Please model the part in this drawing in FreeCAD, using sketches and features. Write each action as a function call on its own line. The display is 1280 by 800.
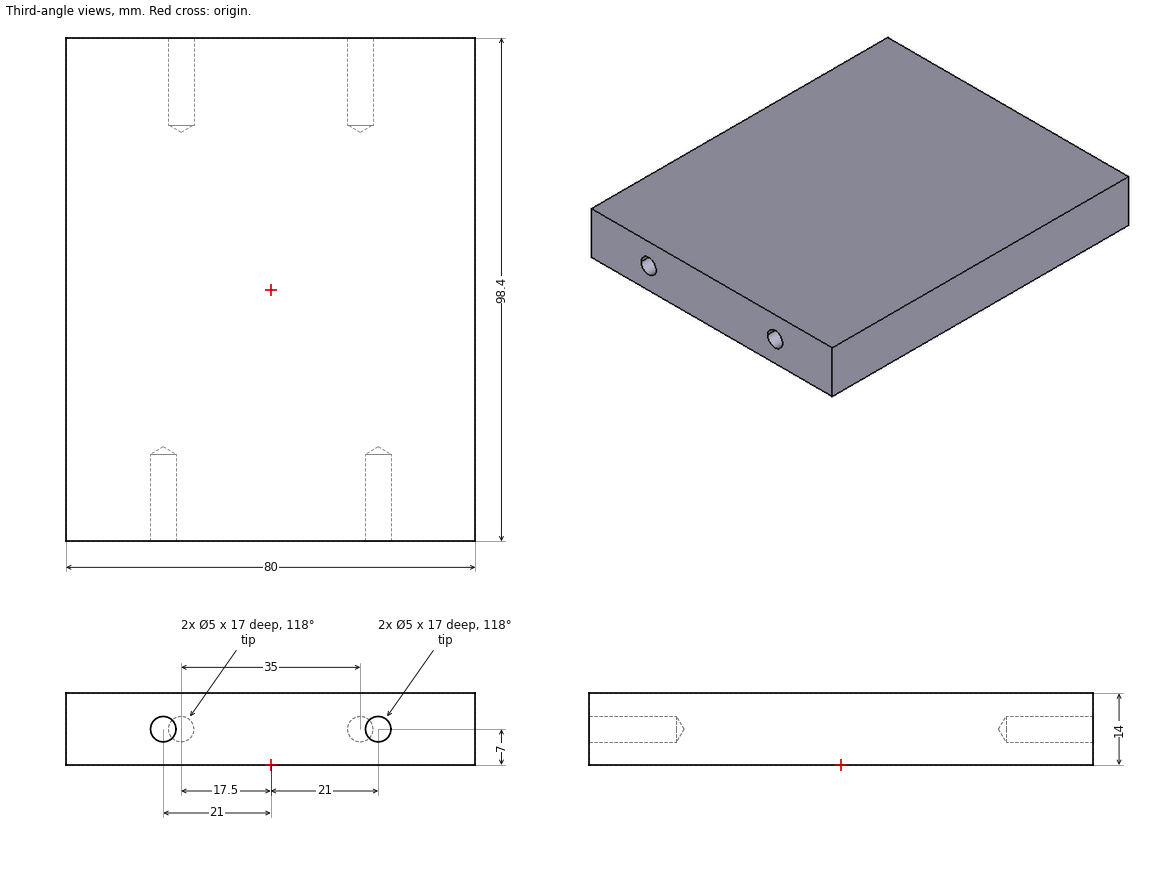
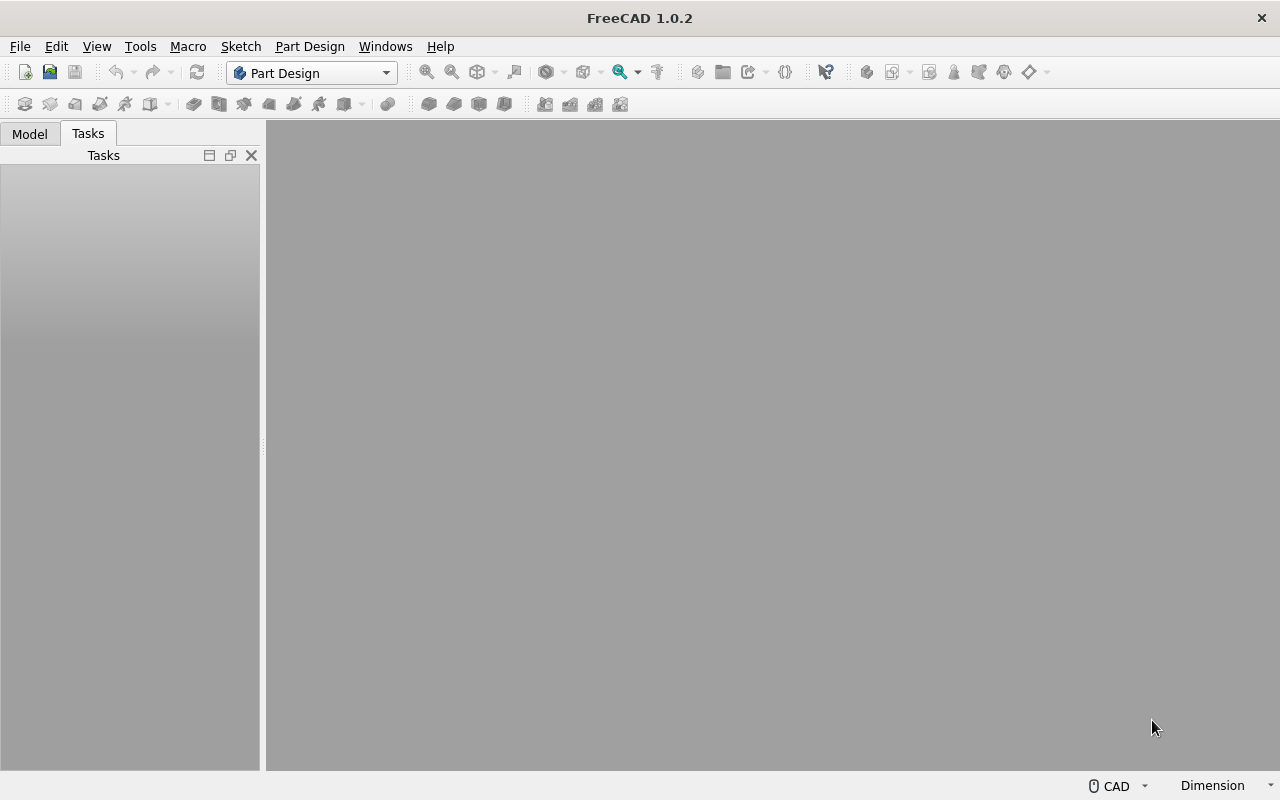
click(25, 72)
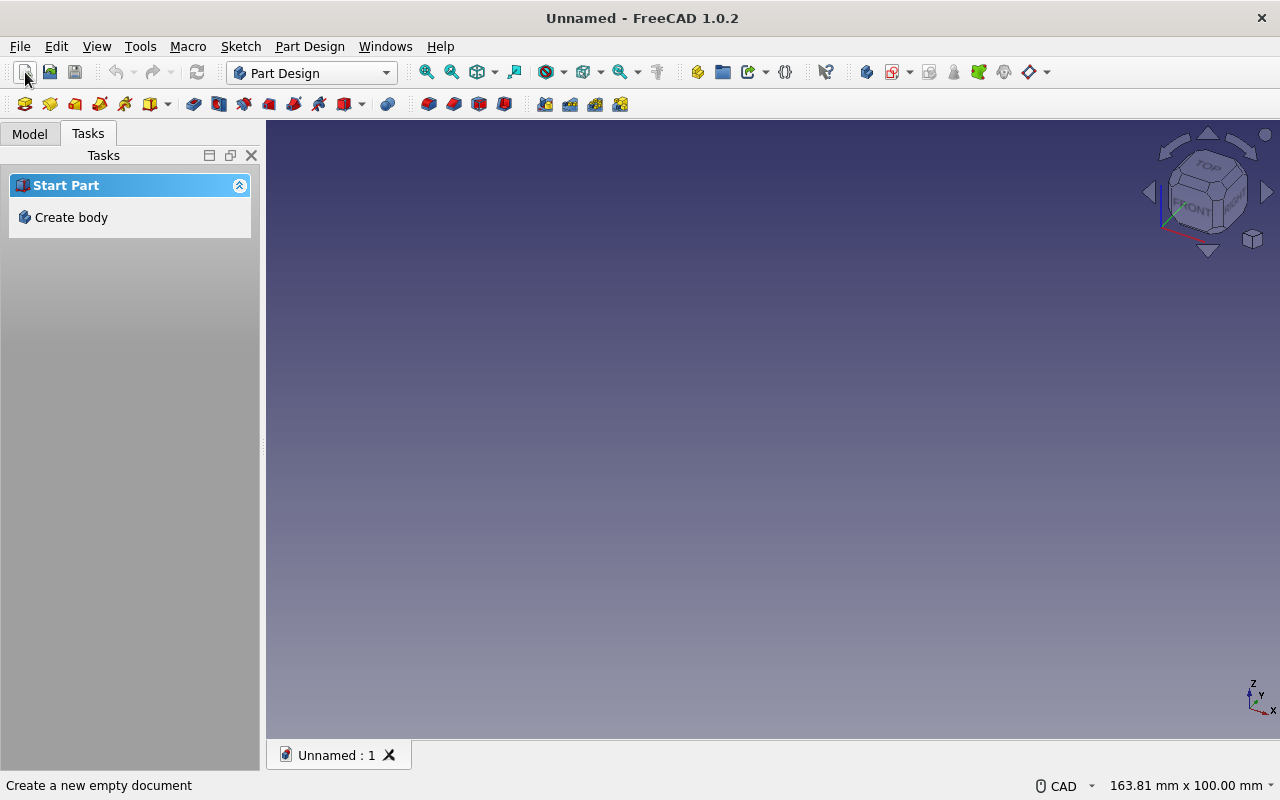
click(892, 72)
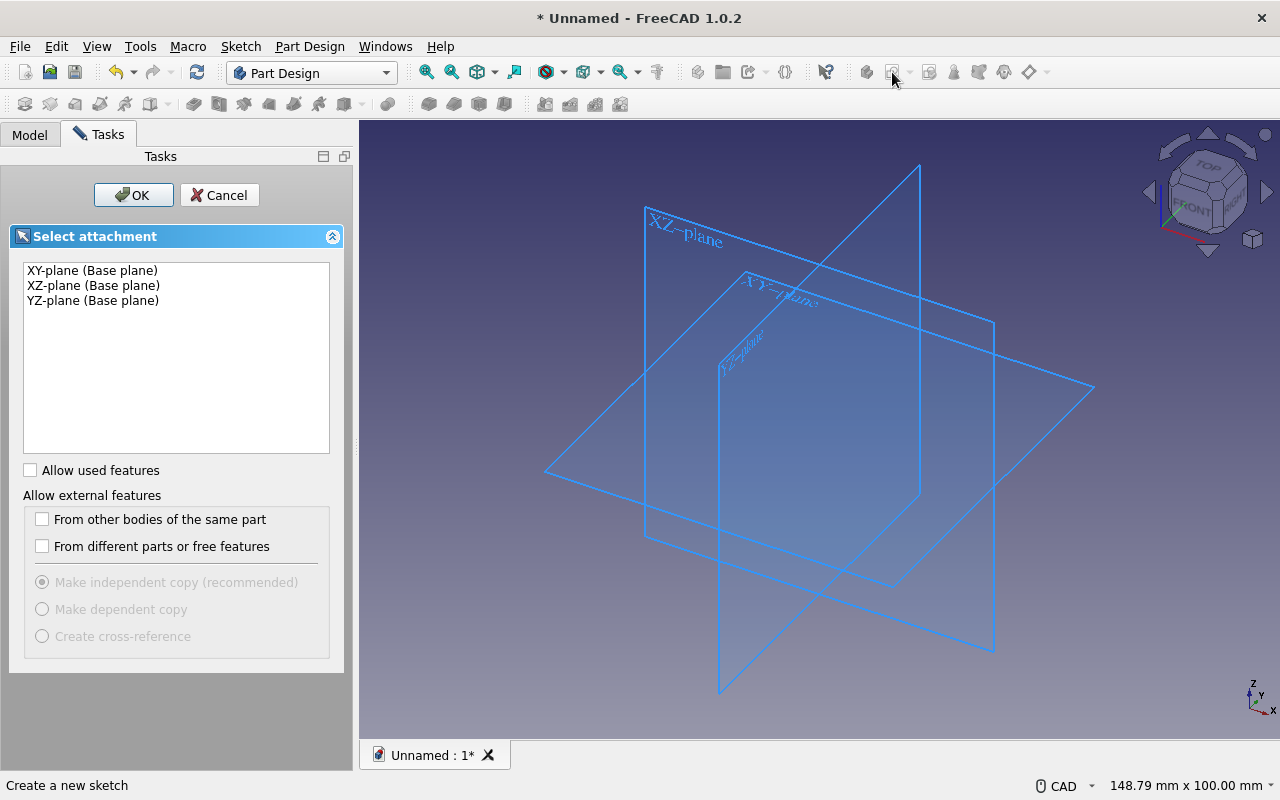
click(84, 270)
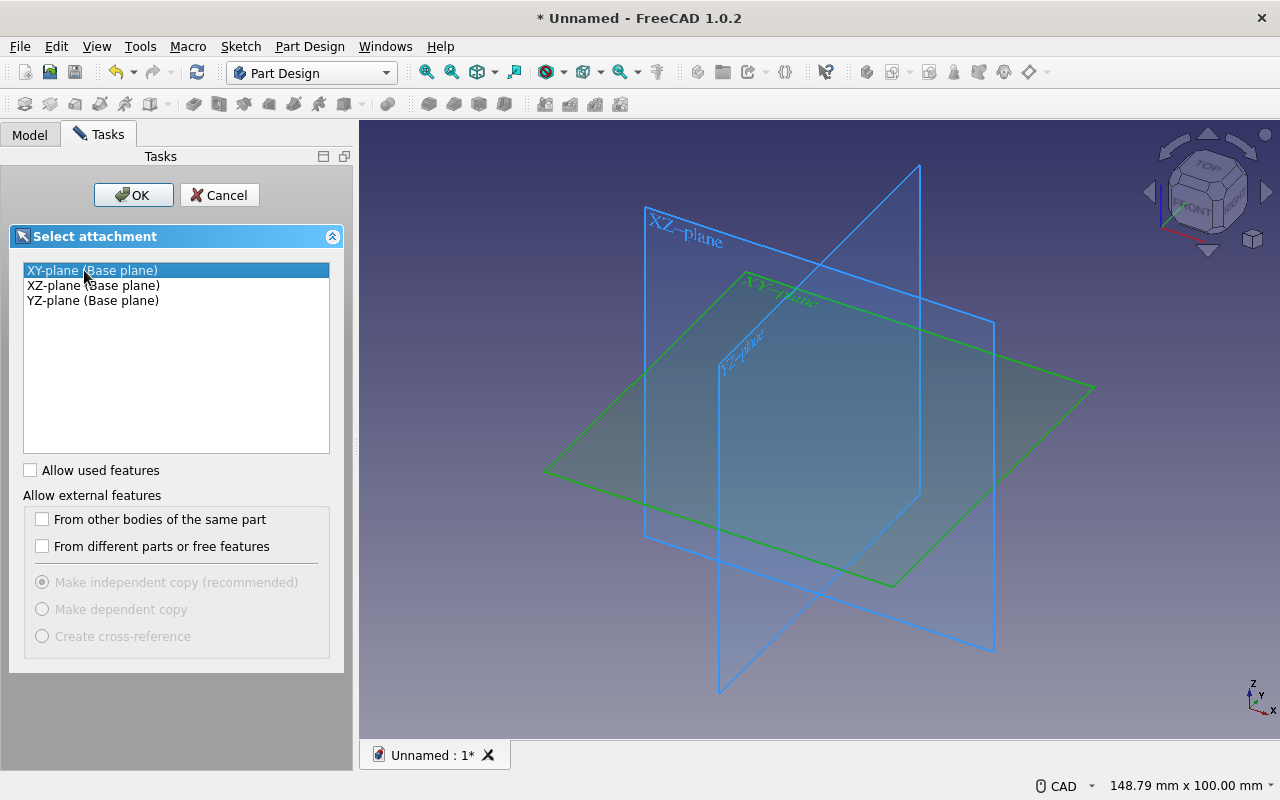
click(134, 195)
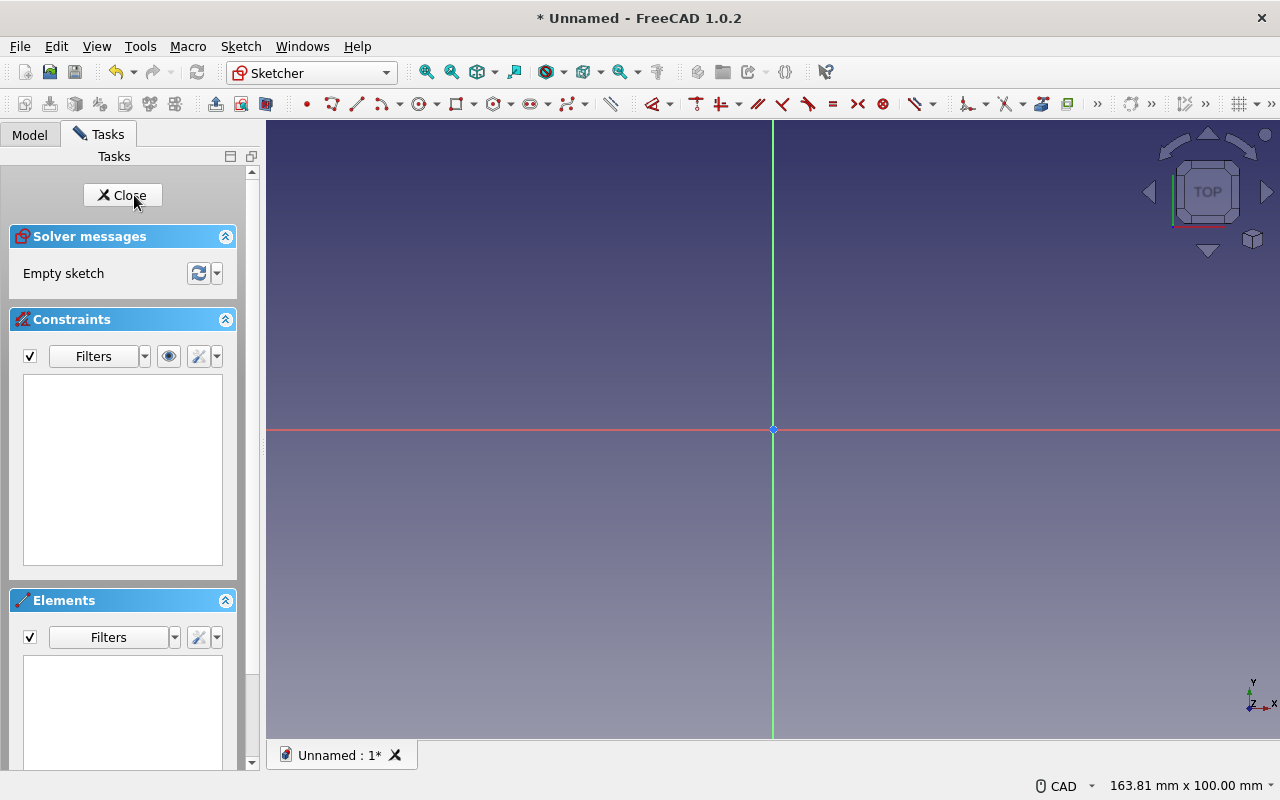
scroll(565, 429, down, 2)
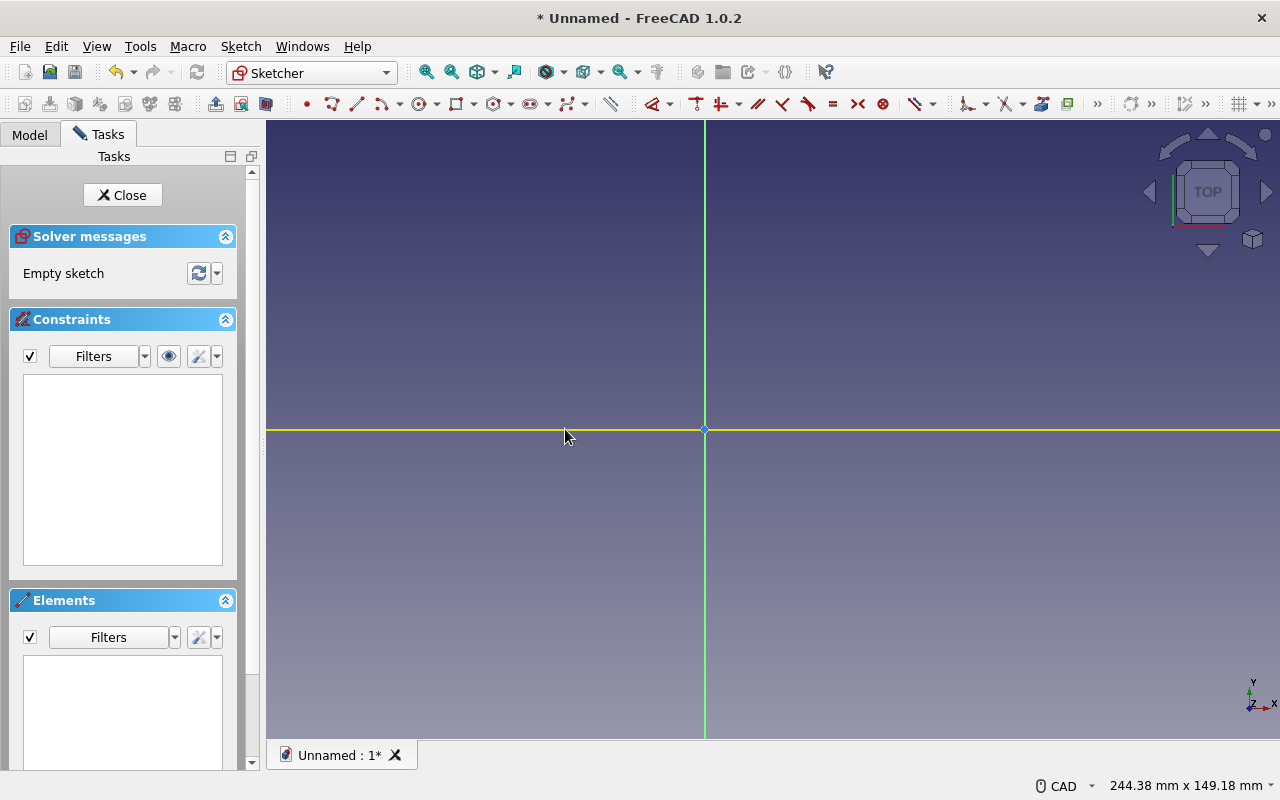
click(474, 104)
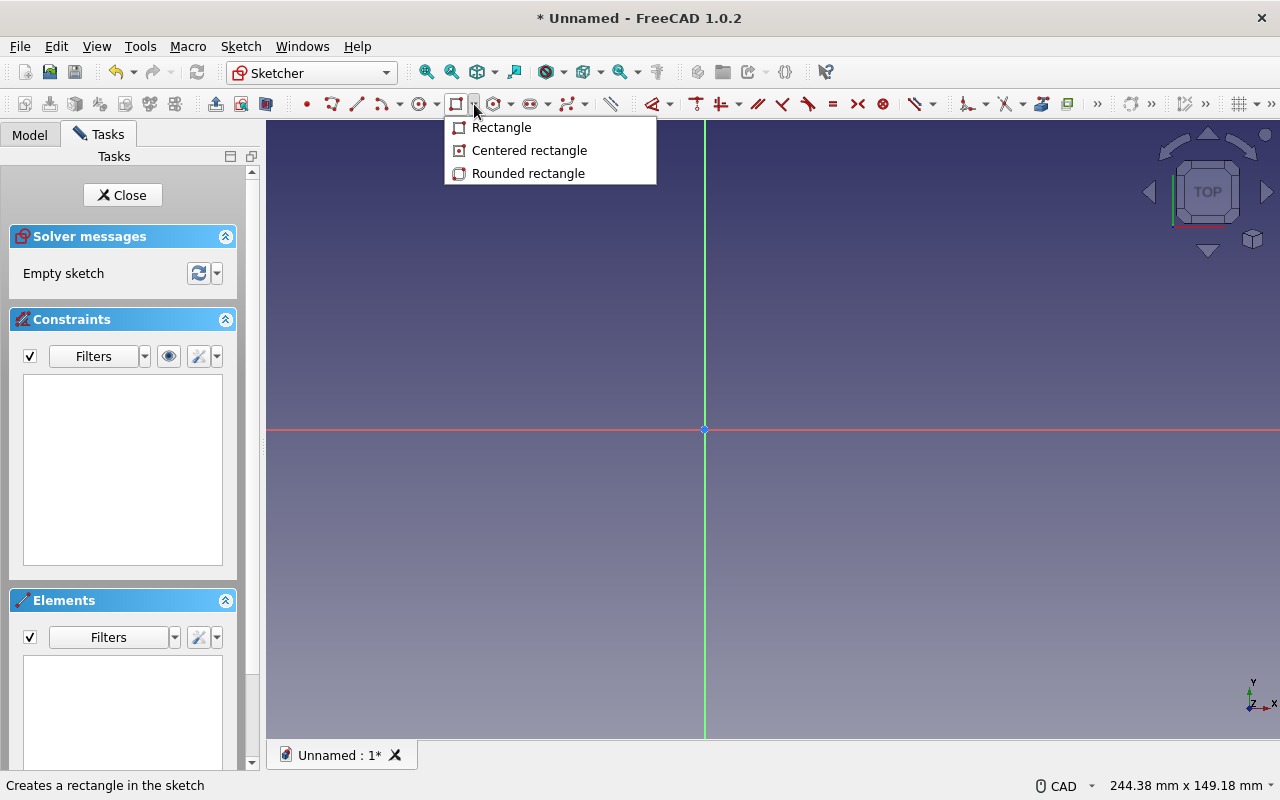
click(550, 150)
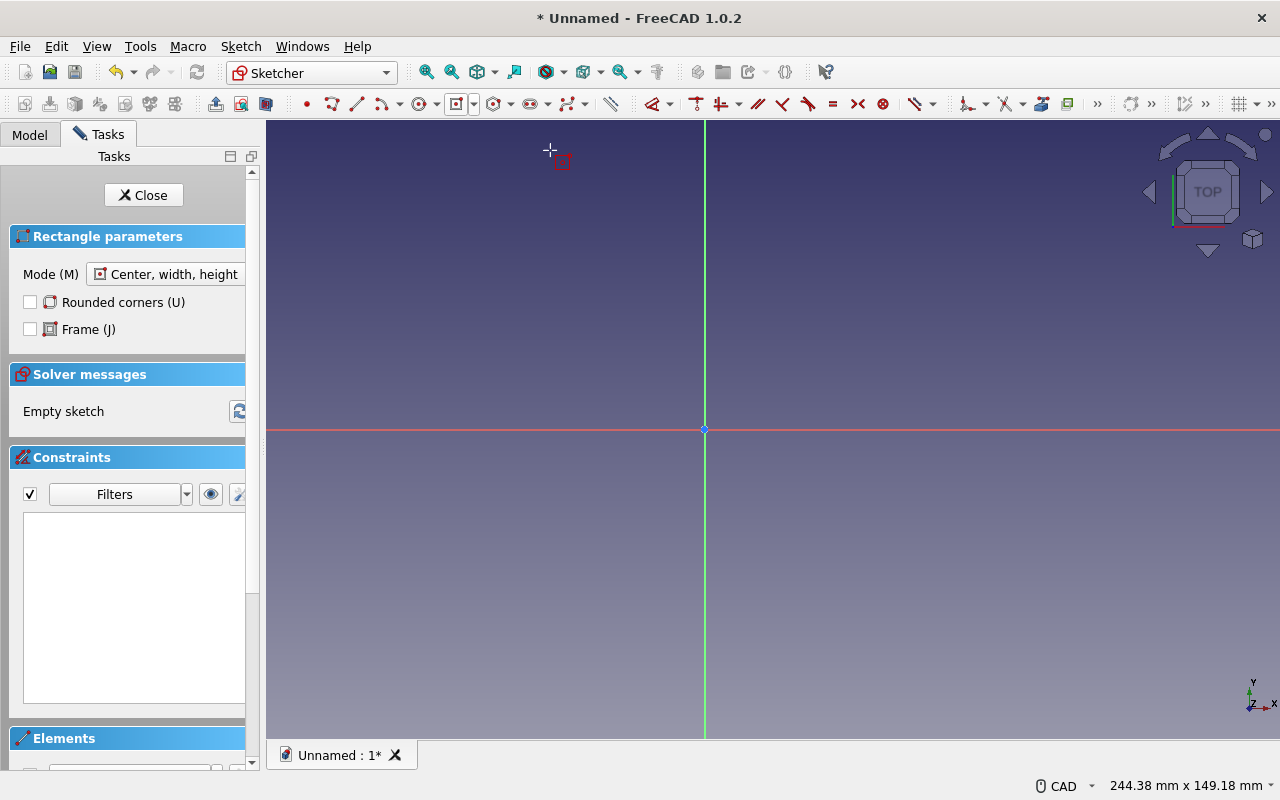
click(705, 430)
click(870, 225)
key(Escape)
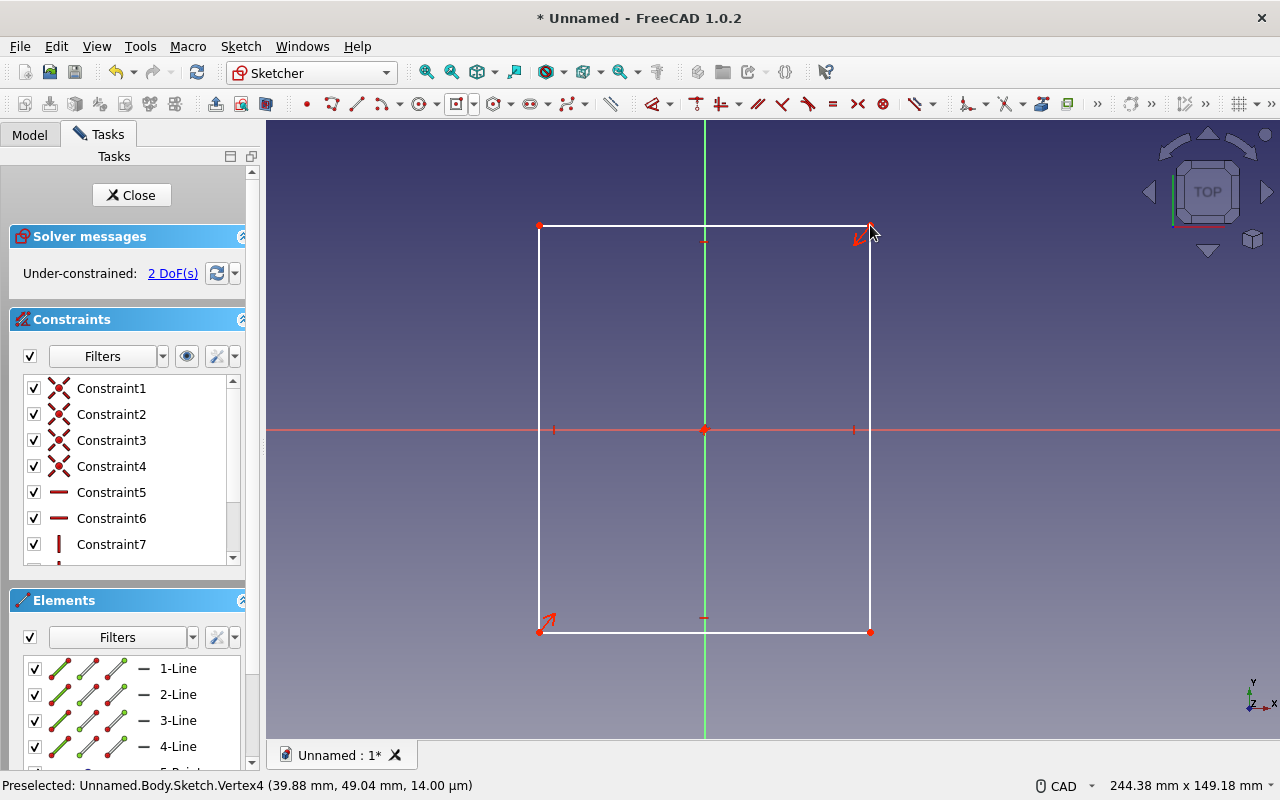
click(652, 104)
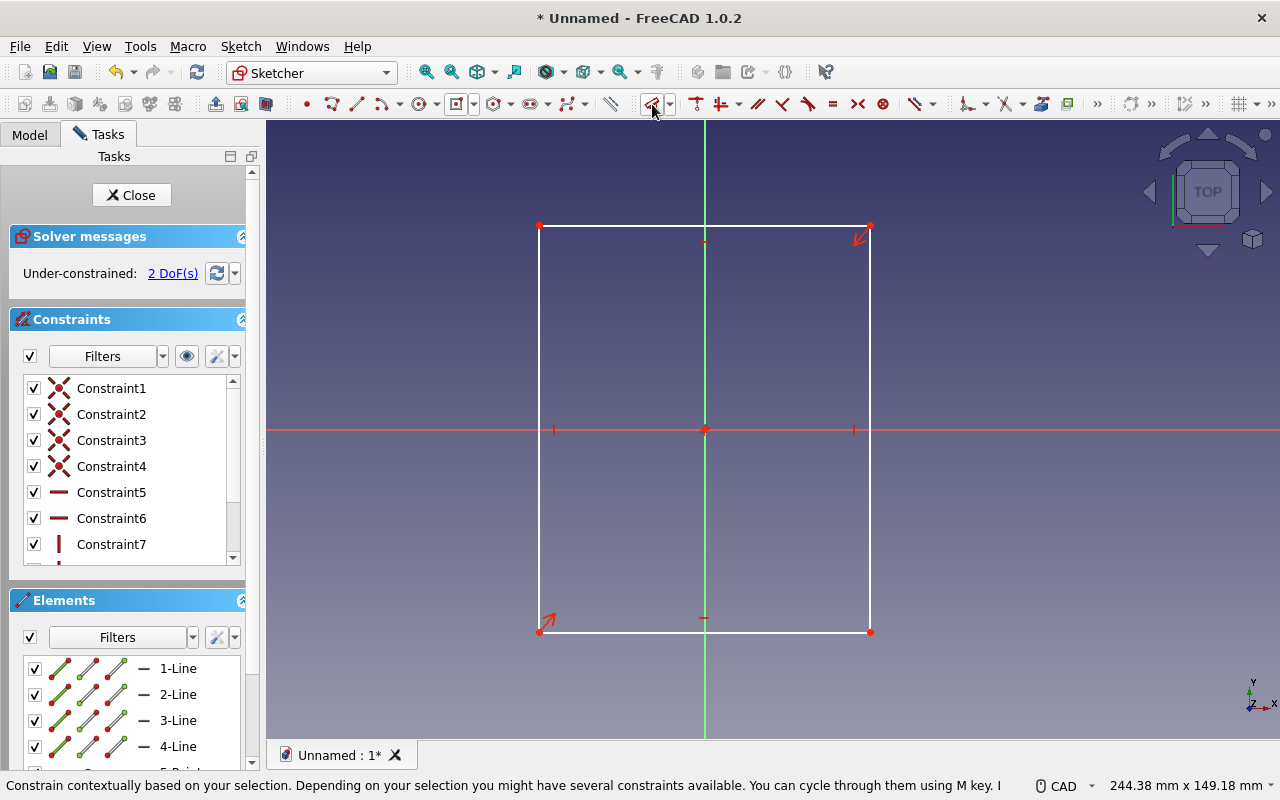
click(638, 633)
click(628, 667)